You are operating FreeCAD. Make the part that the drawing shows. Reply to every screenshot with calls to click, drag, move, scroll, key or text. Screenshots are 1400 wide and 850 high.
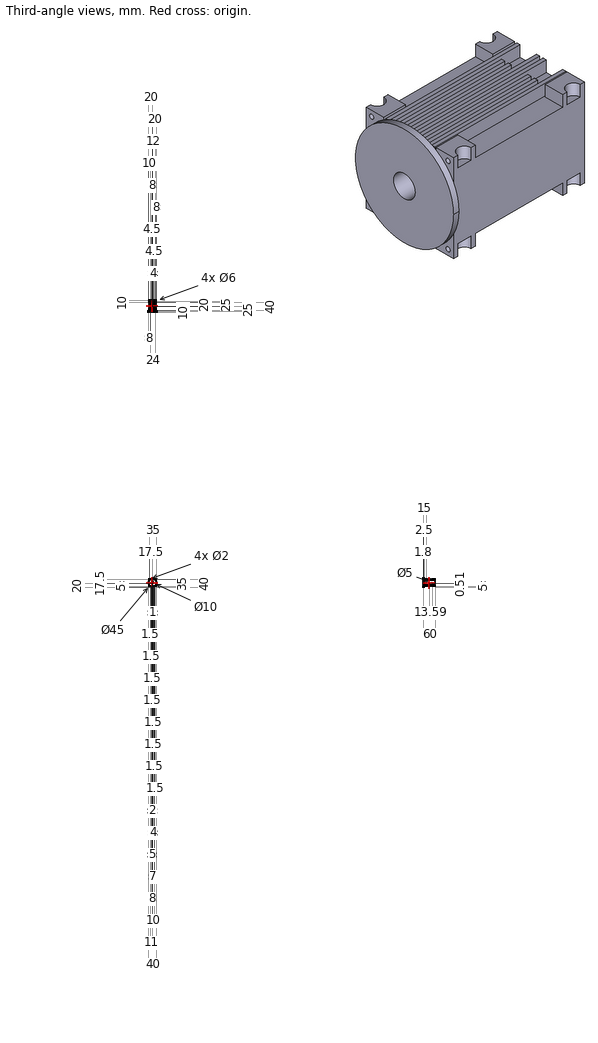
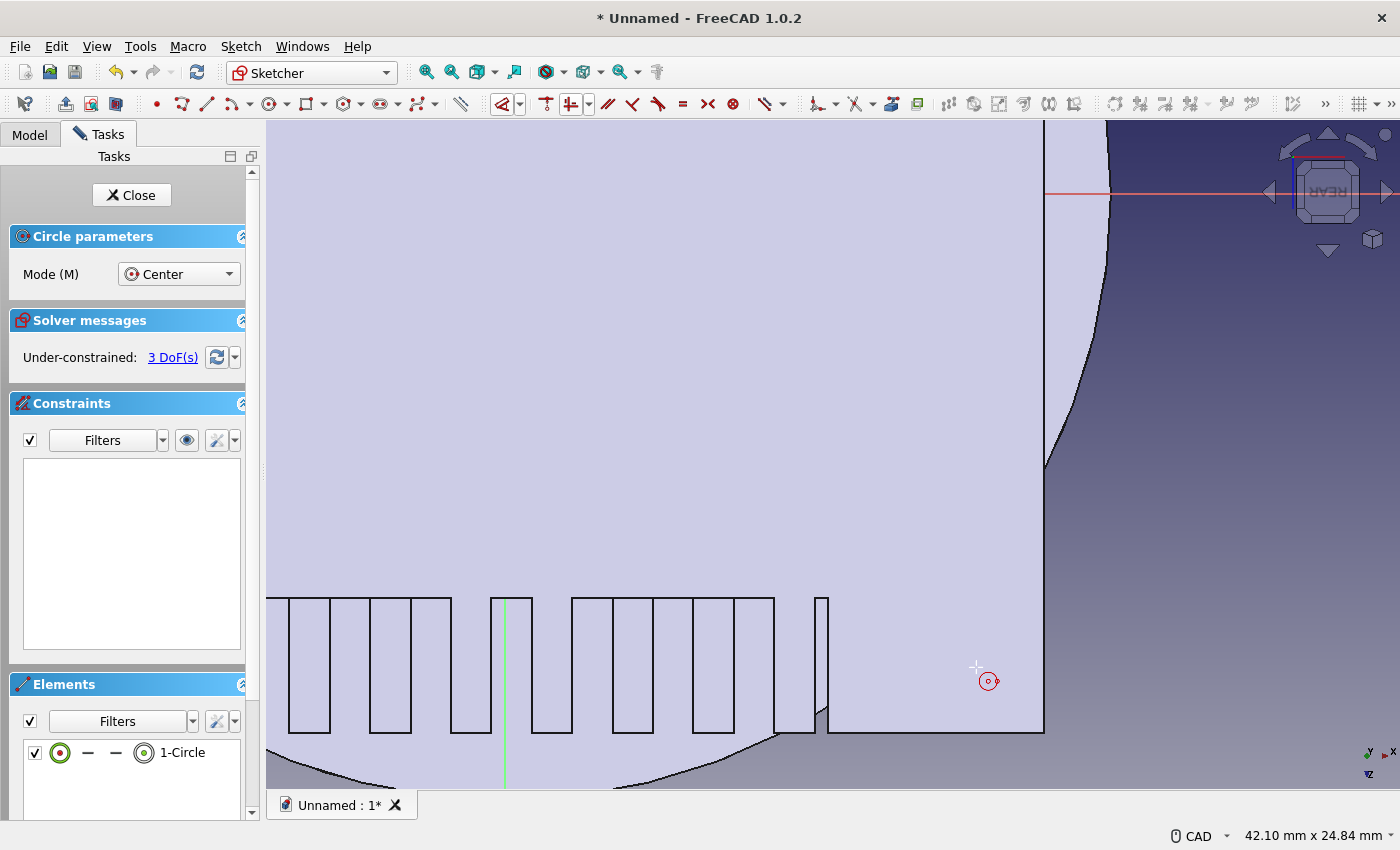
click(976, 665)
click(995, 646)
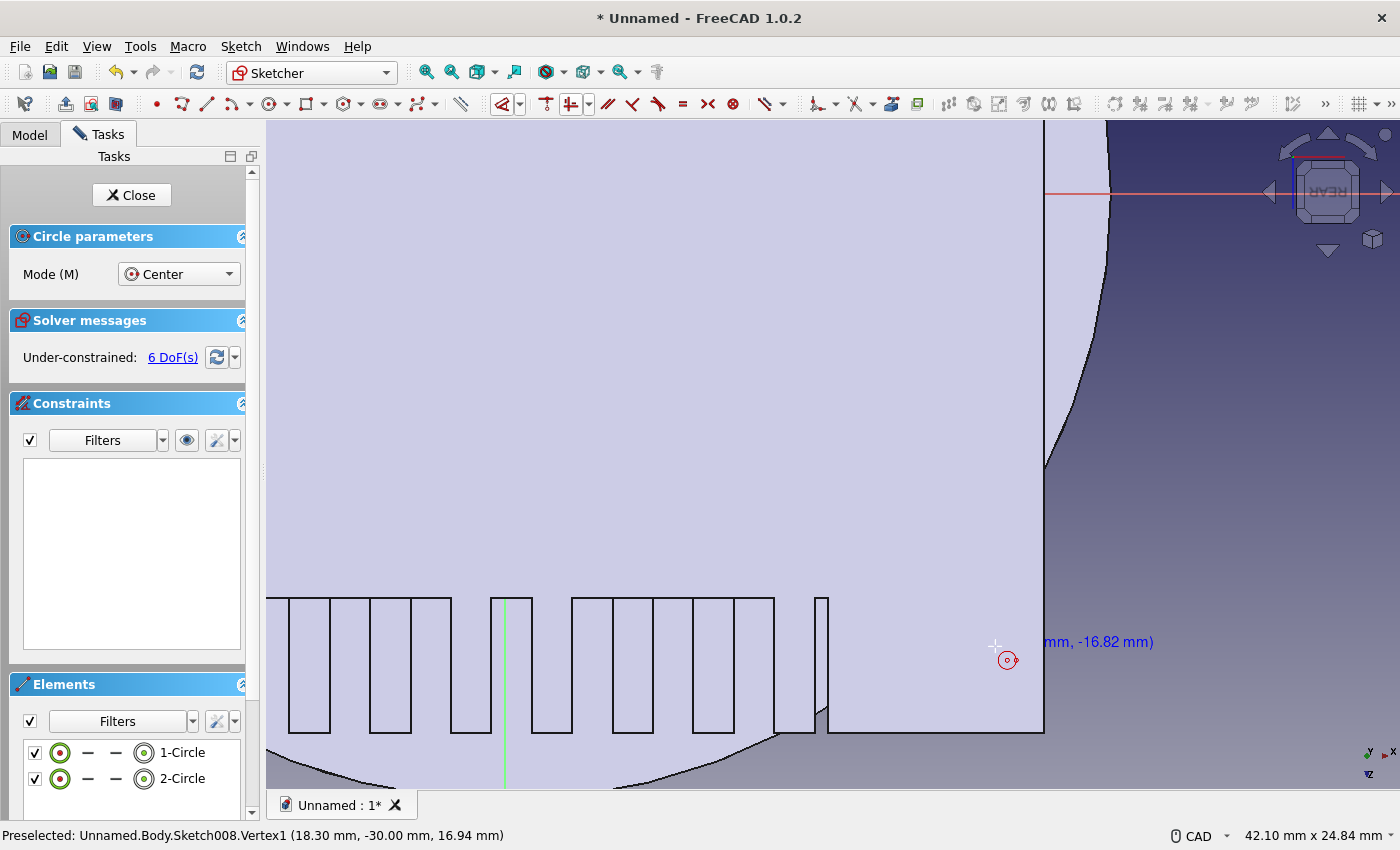
scroll(976, 667, down, 4)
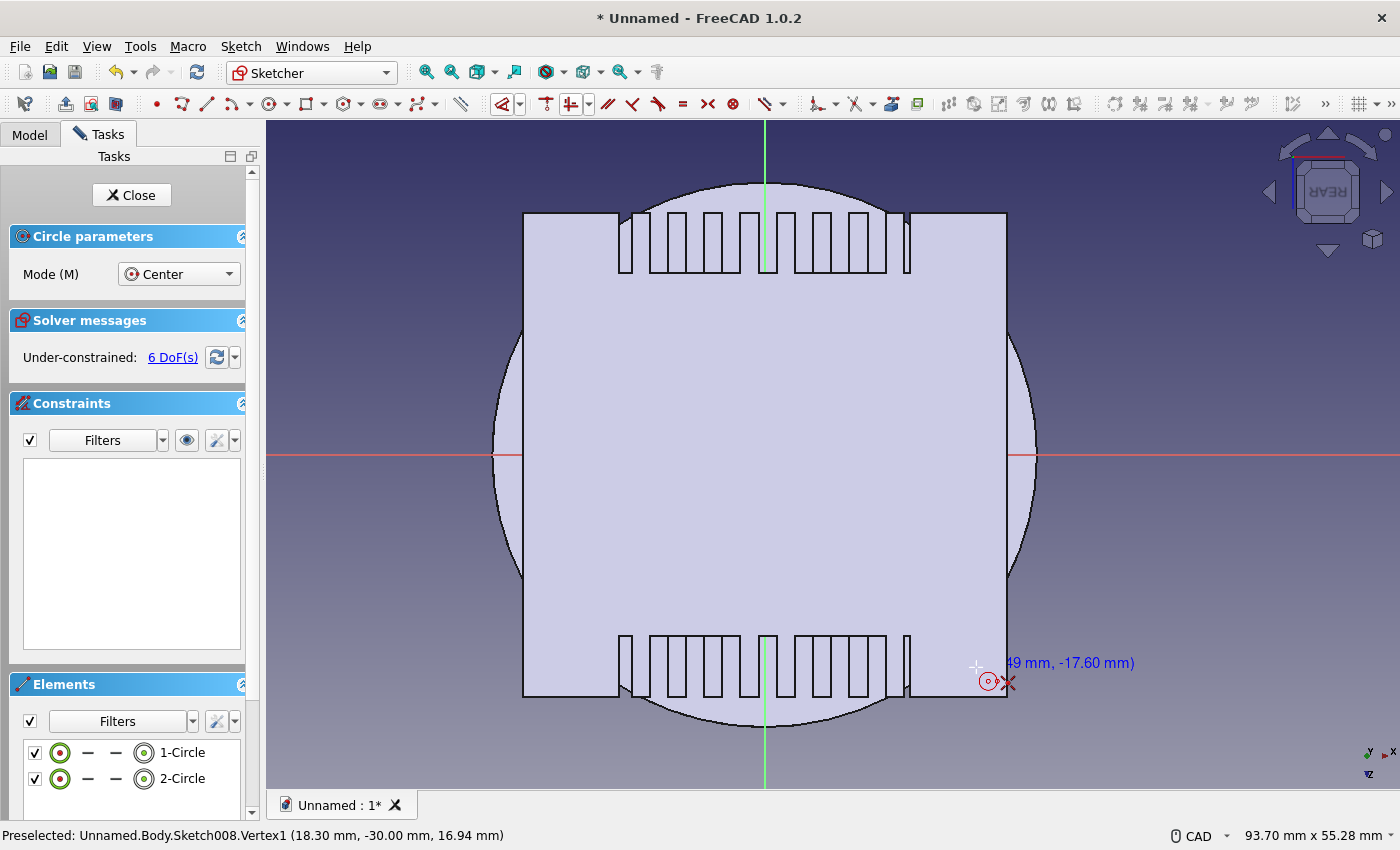
scroll(976, 243, up, 4)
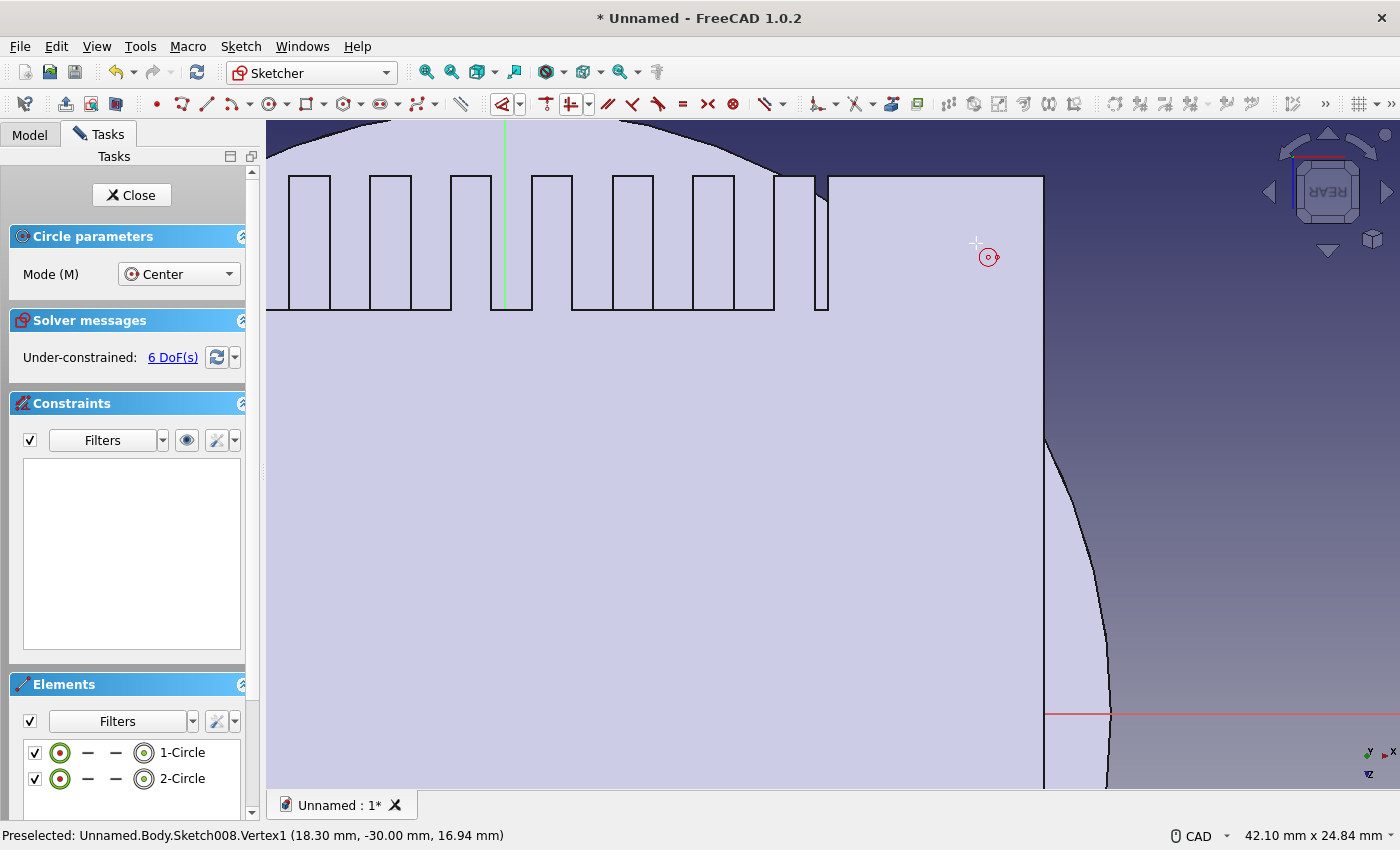
click(976, 243)
click(995, 224)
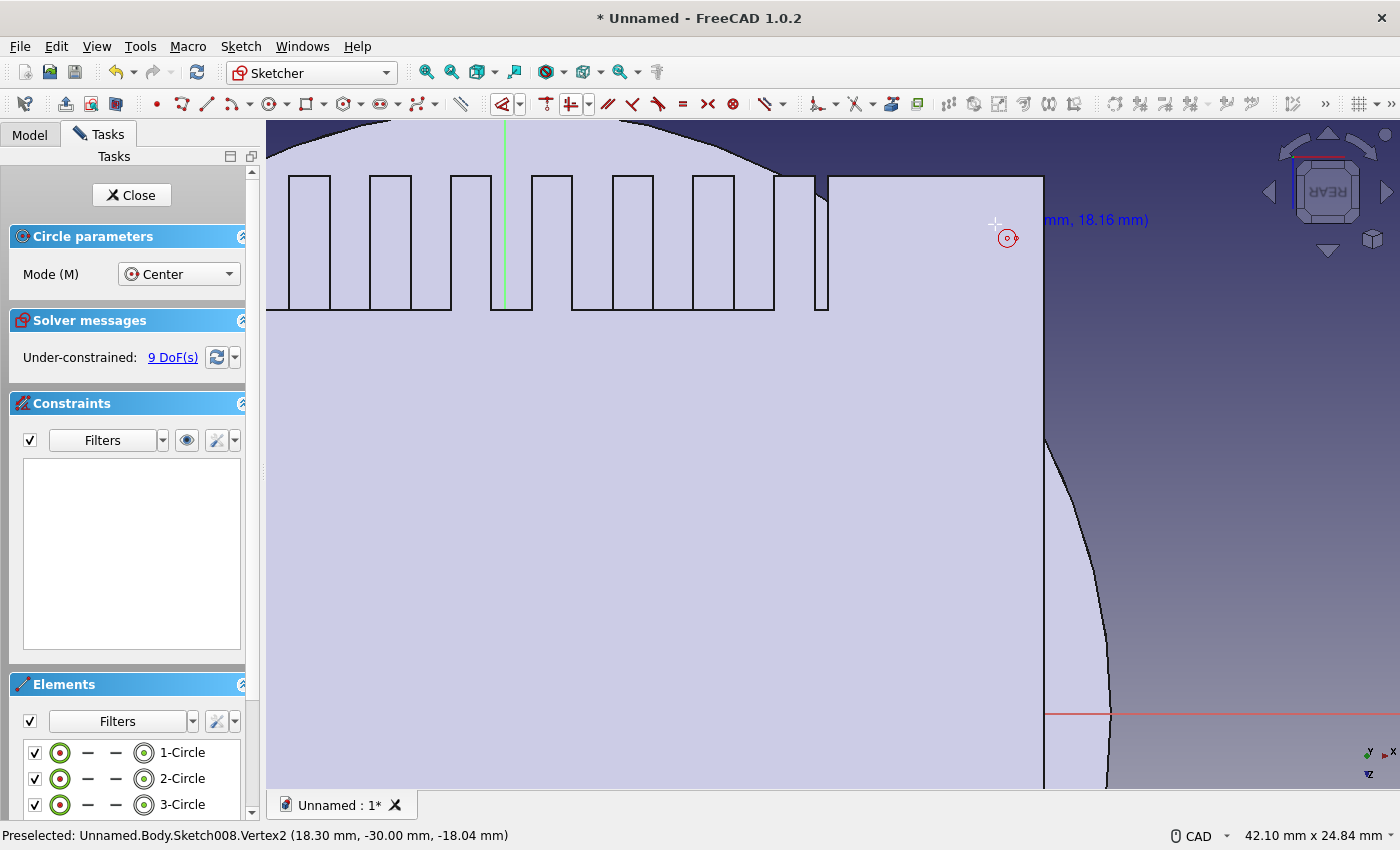
scroll(976, 243, down, 4)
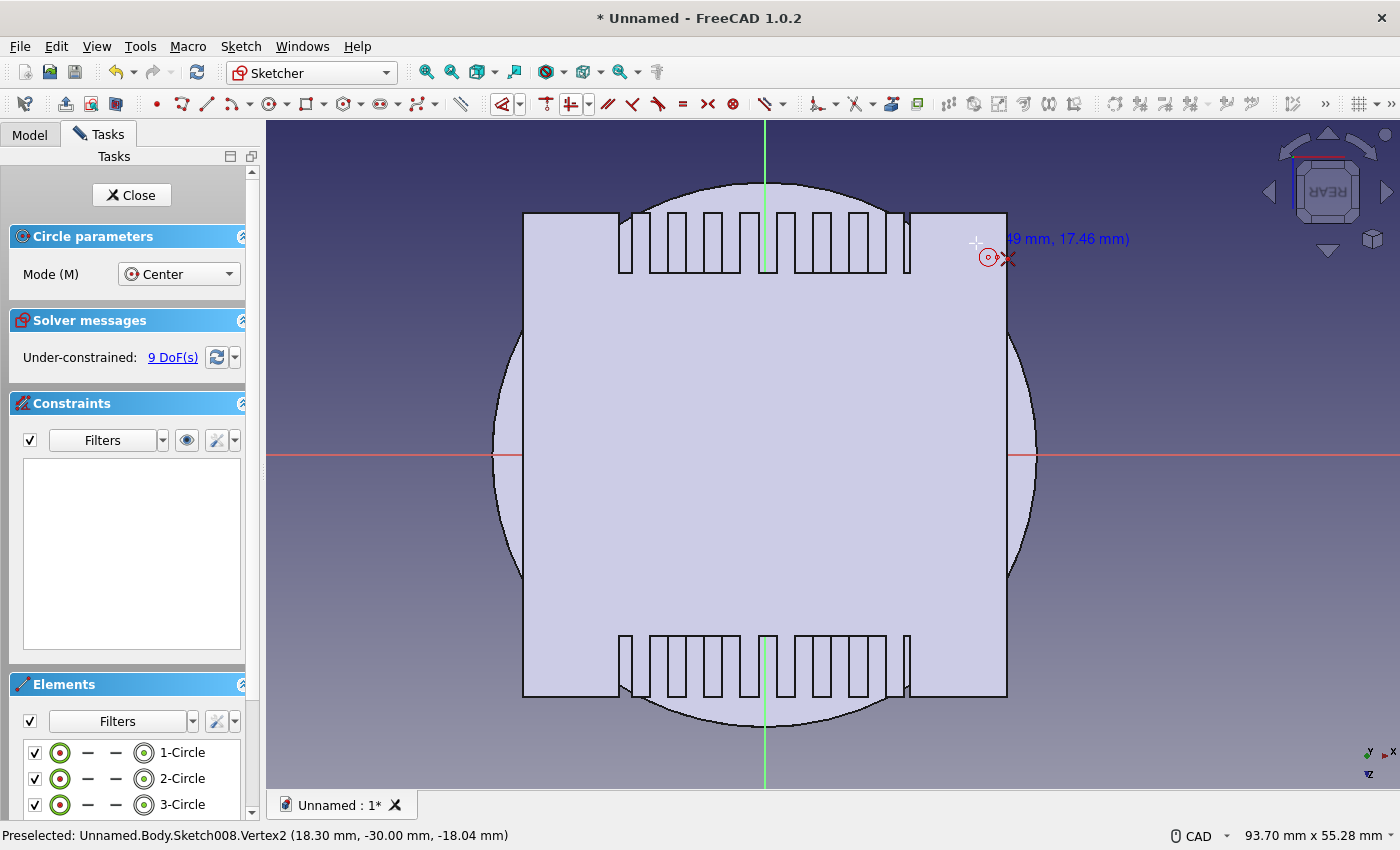
scroll(553, 243, up, 4)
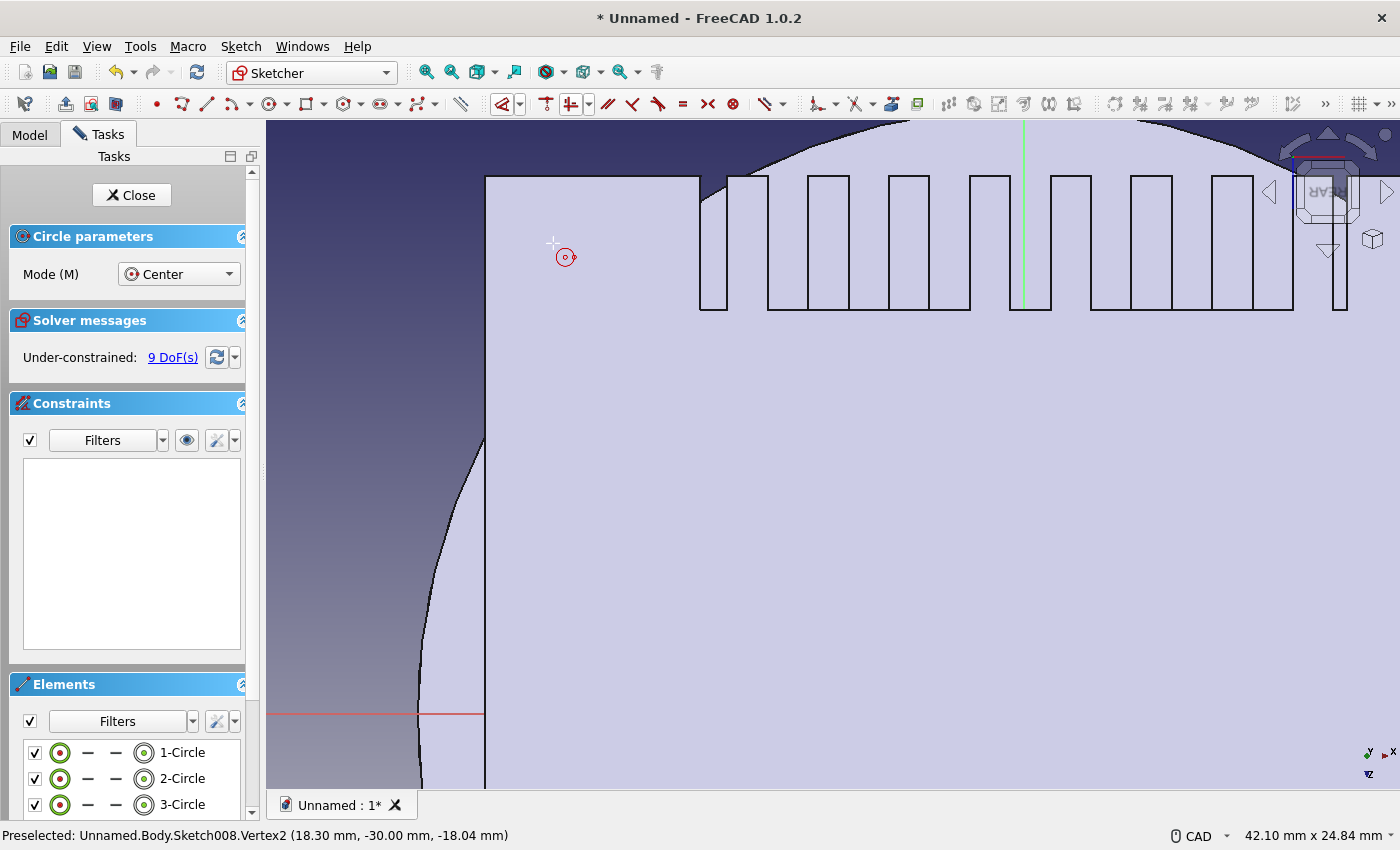
click(552, 243)
click(571, 224)
key(Escape)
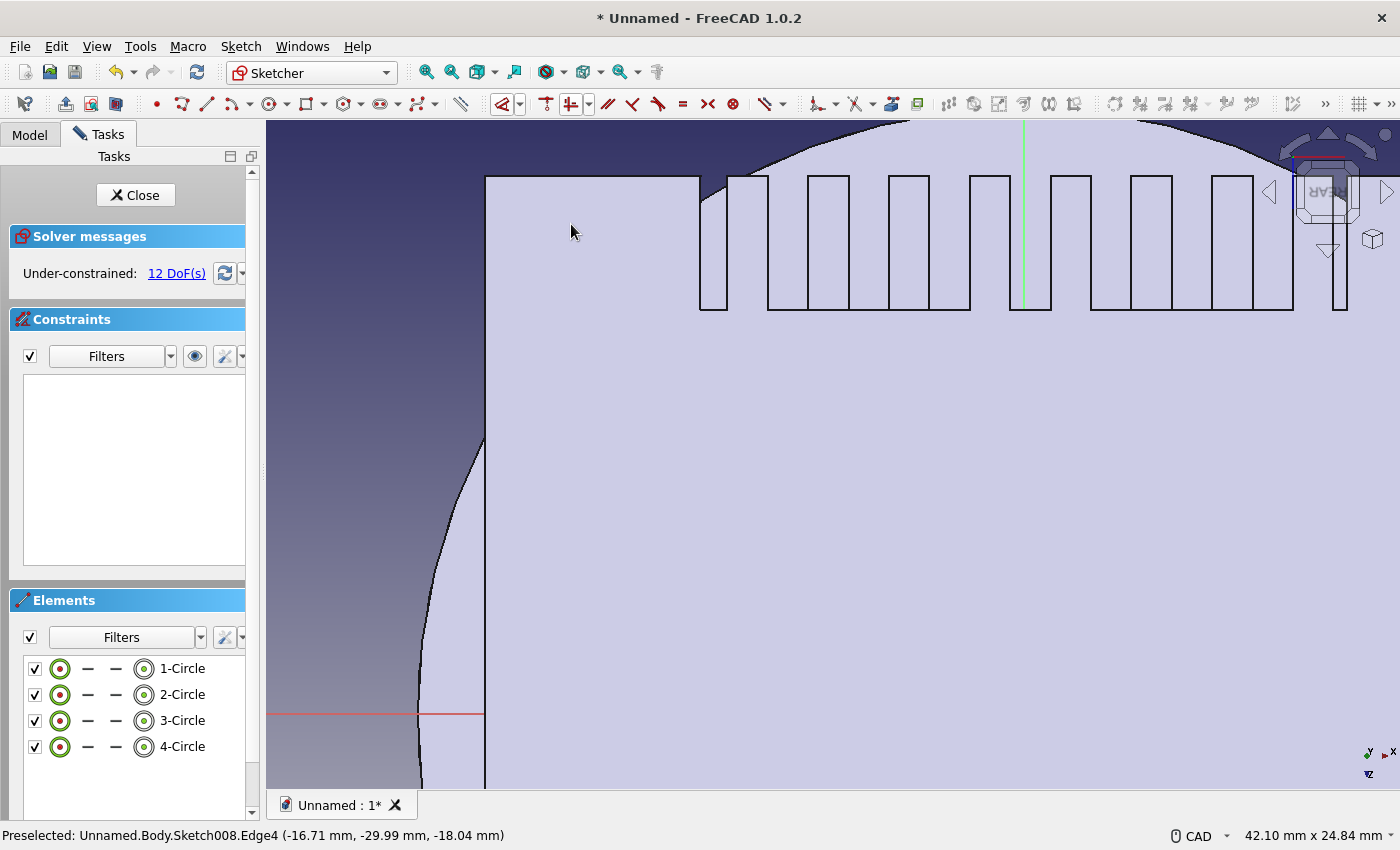
scroll(553, 243, down, 4)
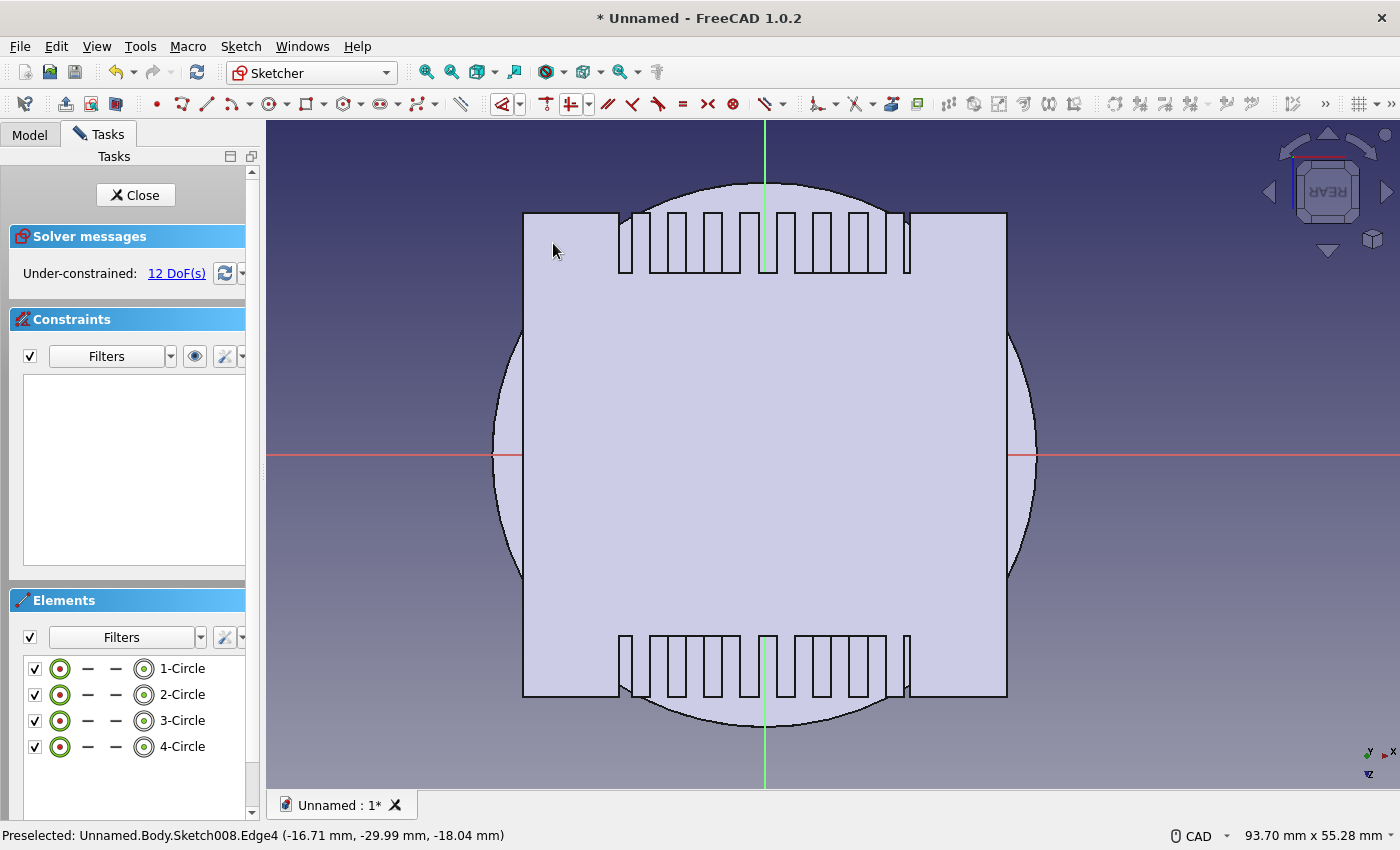
click(561, 658)